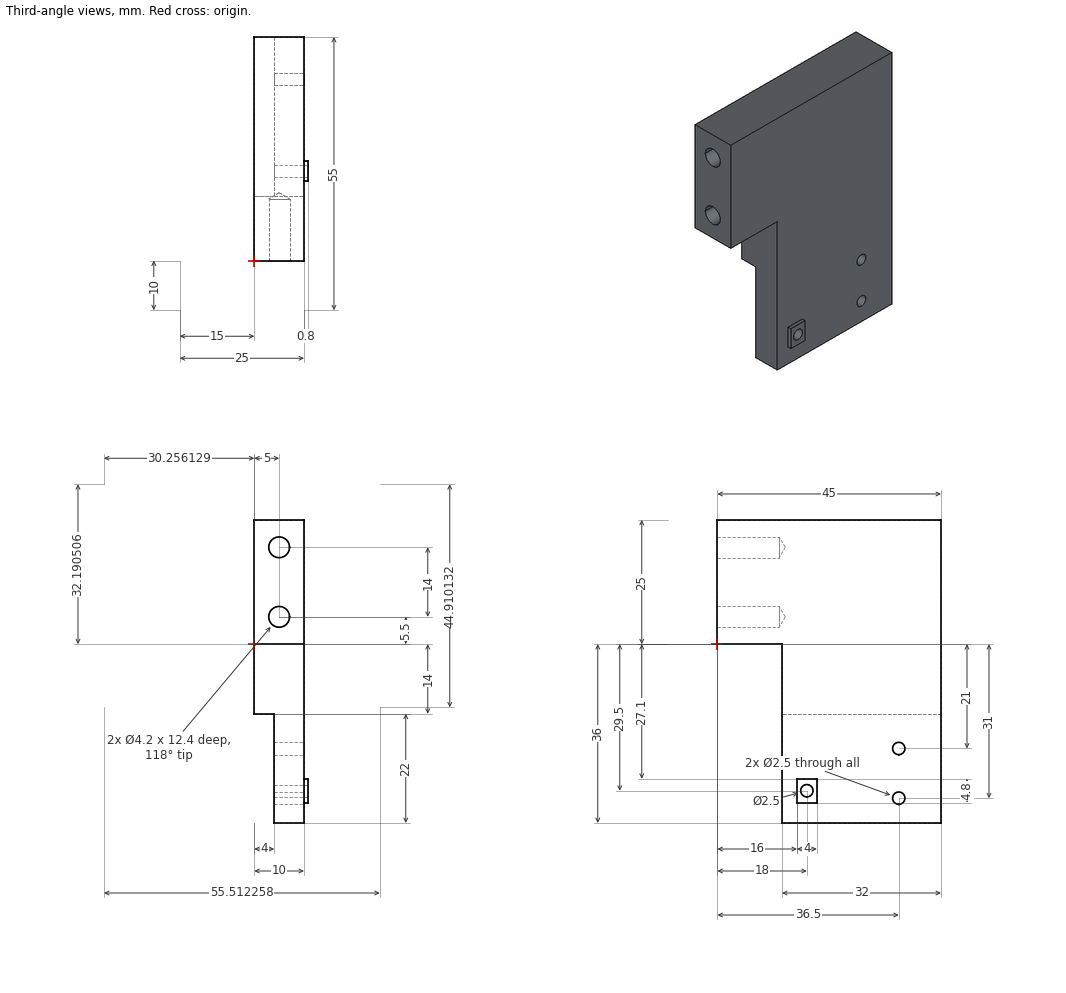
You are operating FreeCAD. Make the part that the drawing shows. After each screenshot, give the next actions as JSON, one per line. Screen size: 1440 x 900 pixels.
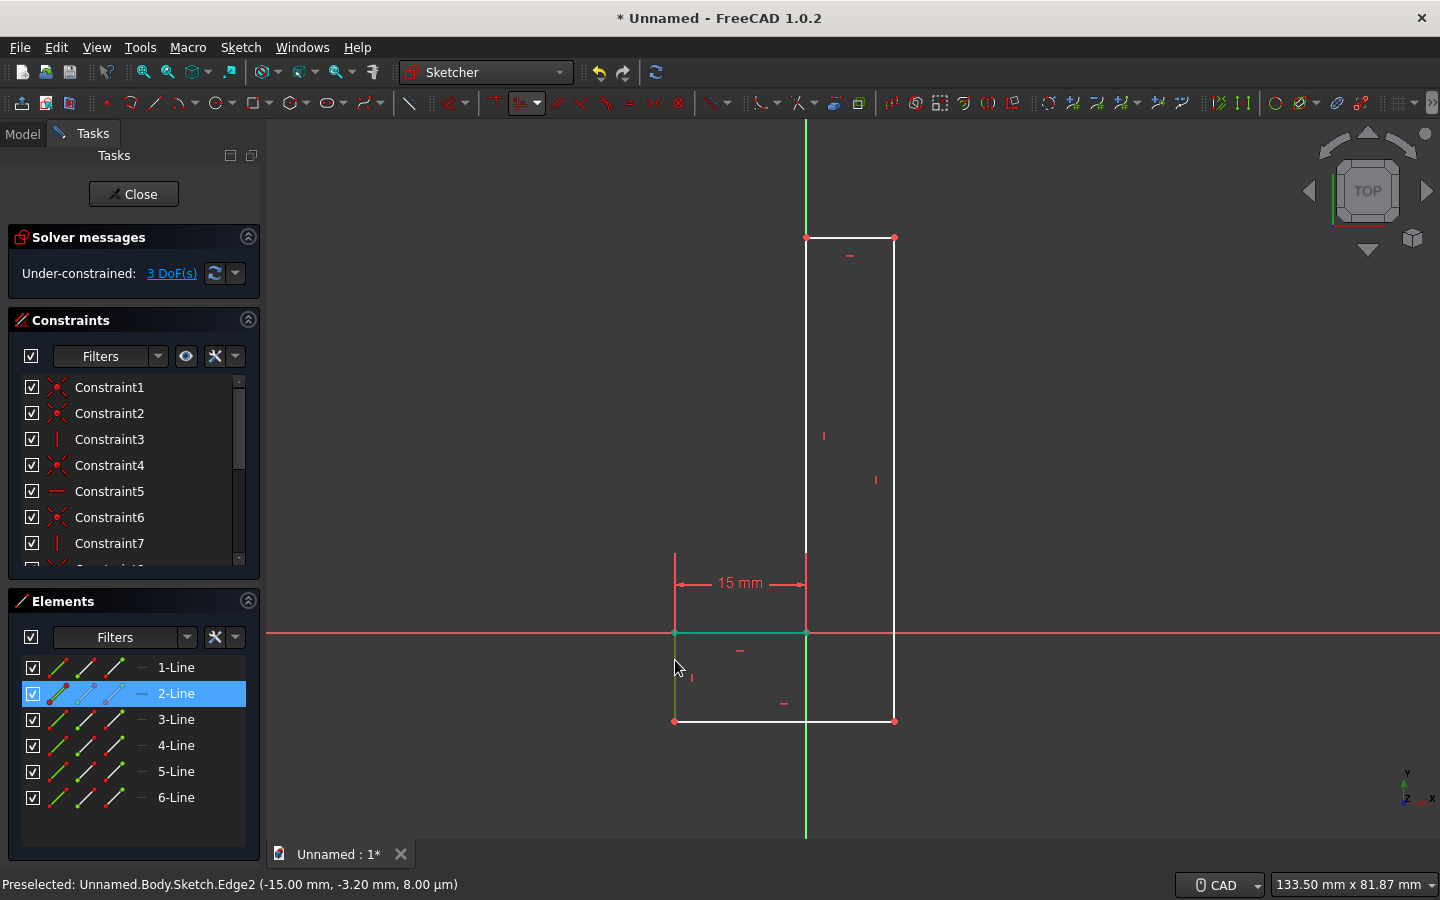
{"action": "key", "text": "i"}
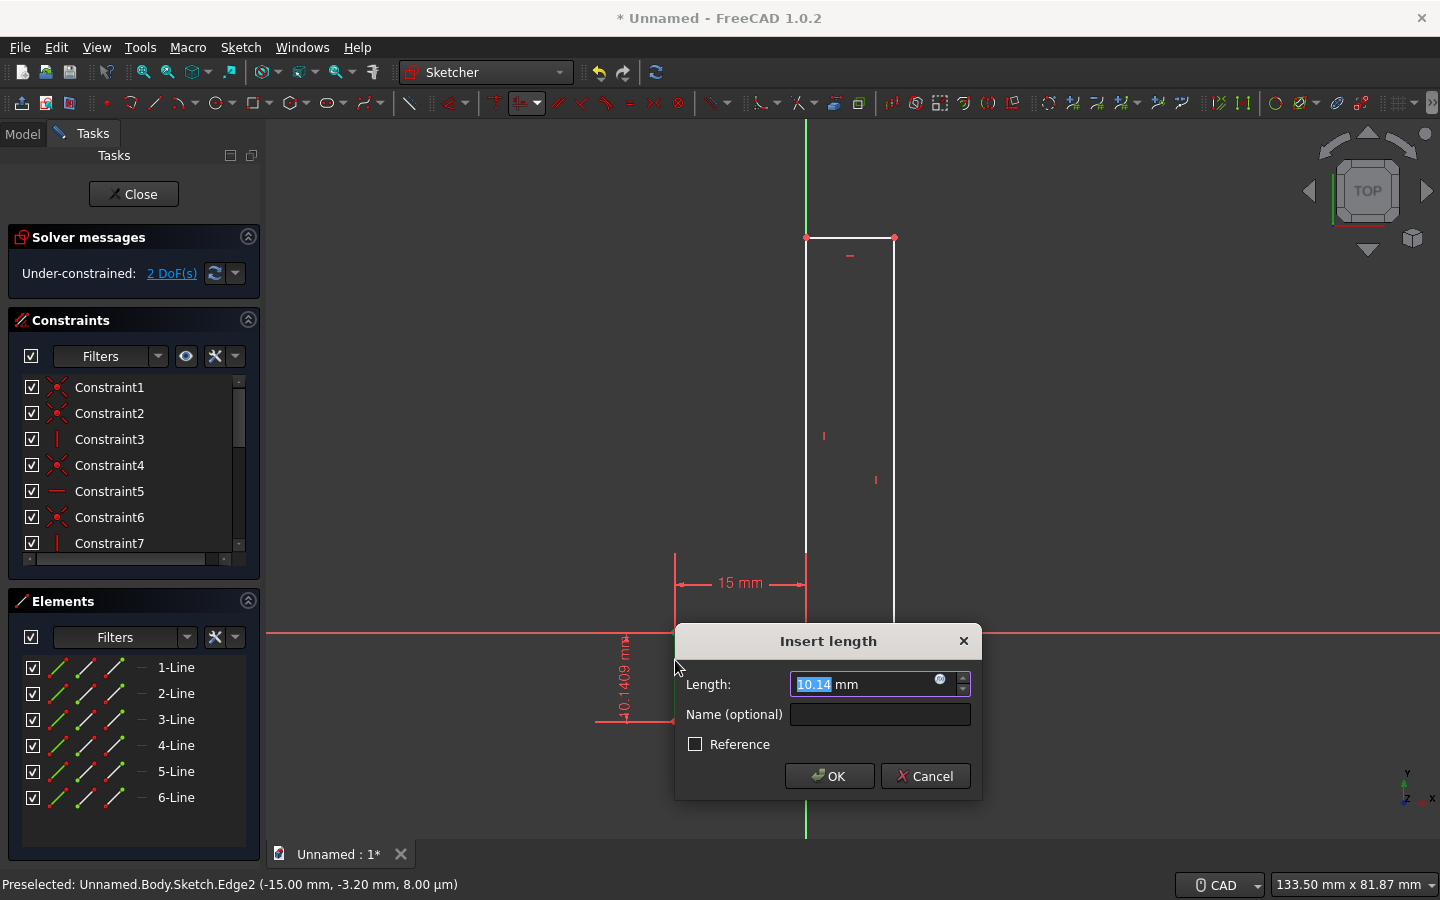
{"action": "type", "text": "10"}
{"action": "key", "text": "Return"}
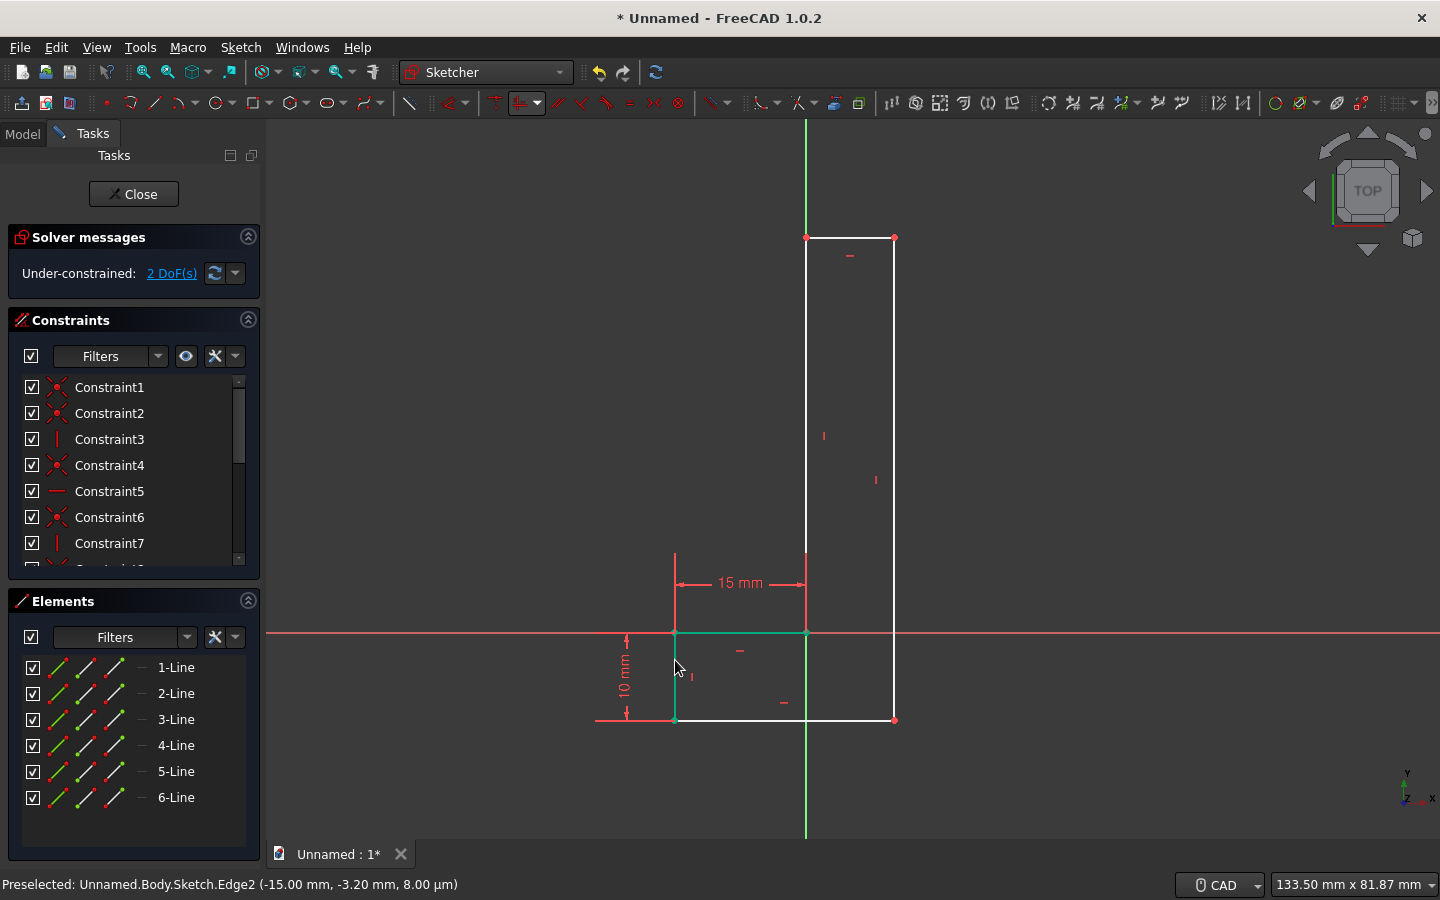
{"action": "left_click", "coordinate": [740, 721]}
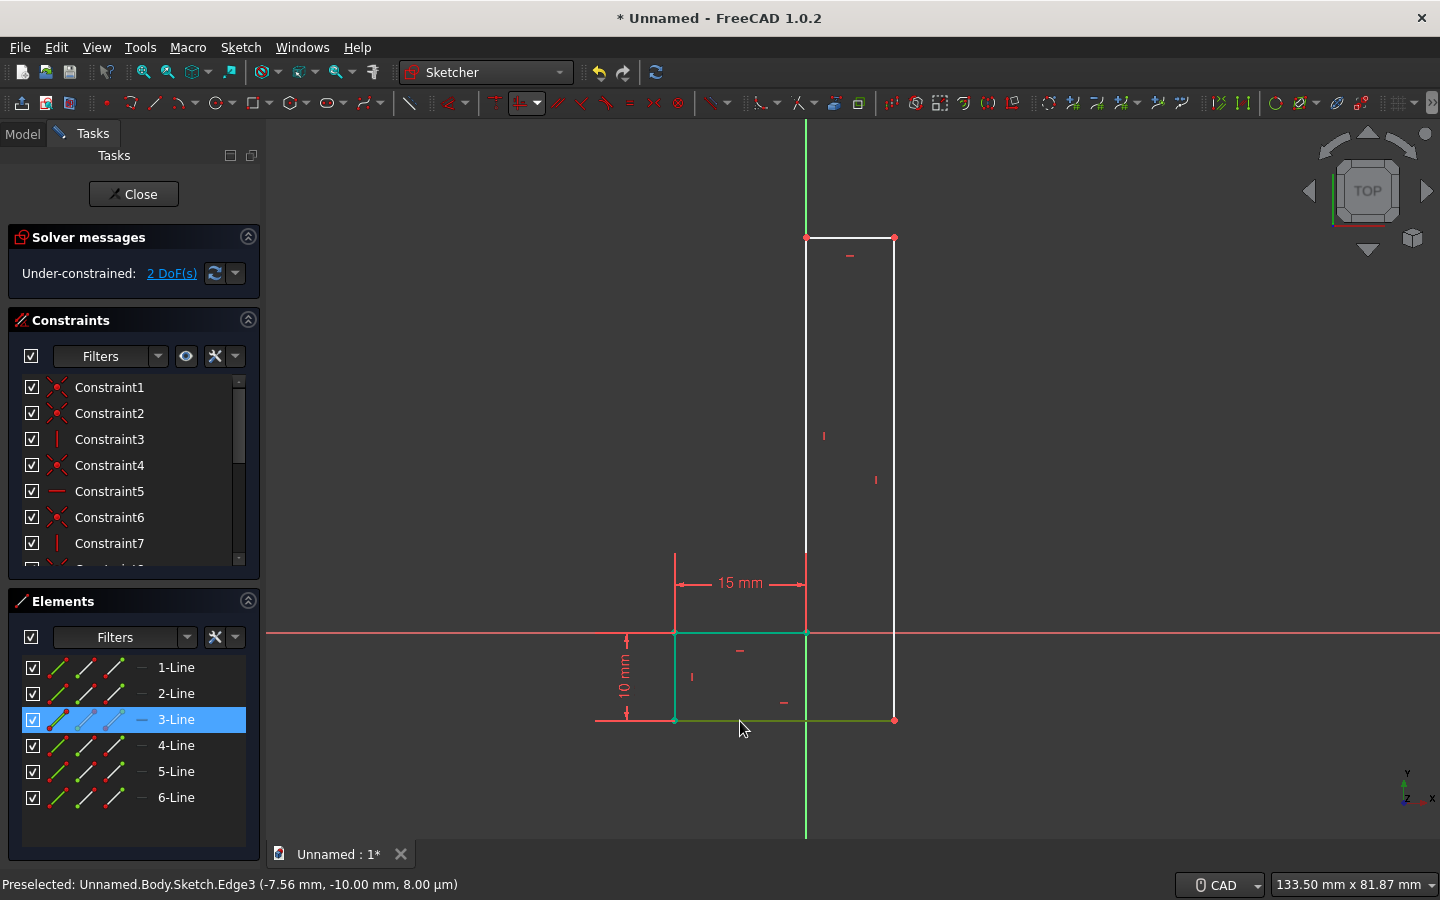
{"action": "key", "text": "l"}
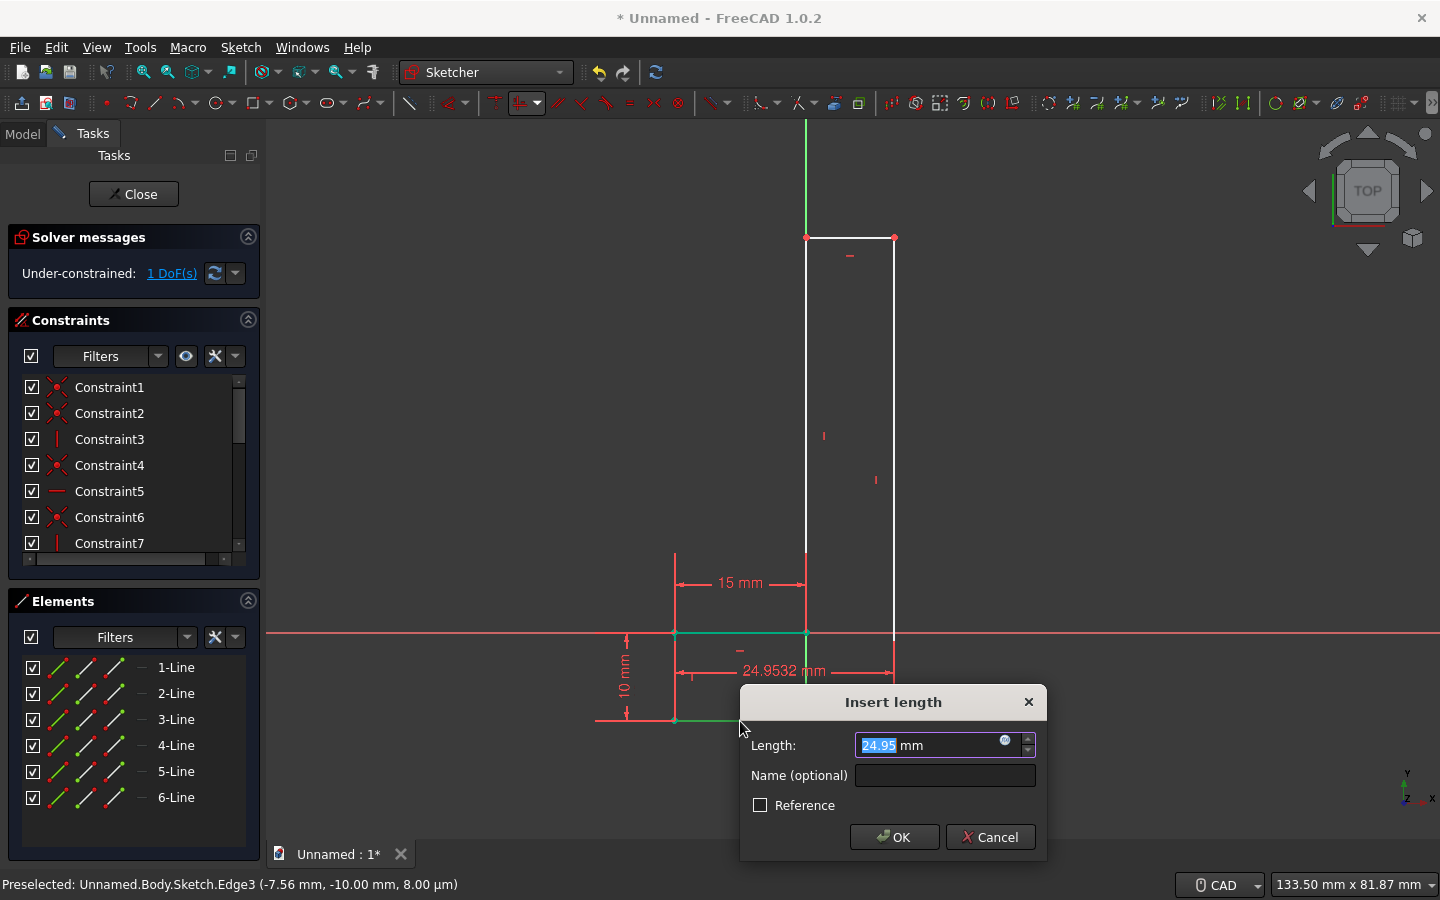
{"action": "type", "text": "25"}
{"action": "key", "text": "Return"}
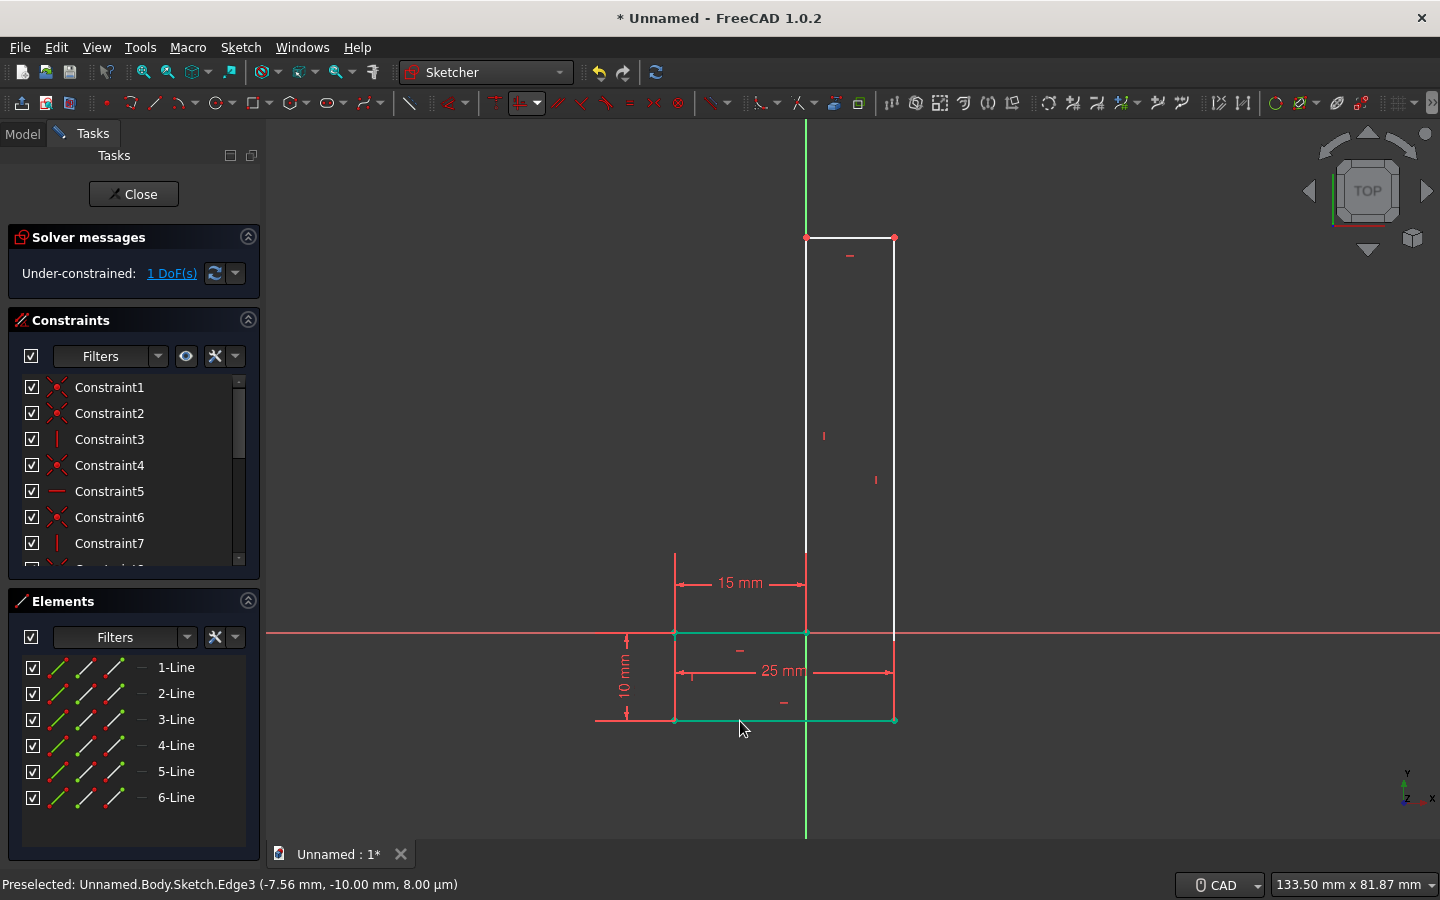
{"action": "left_click", "coordinate": [894, 576]}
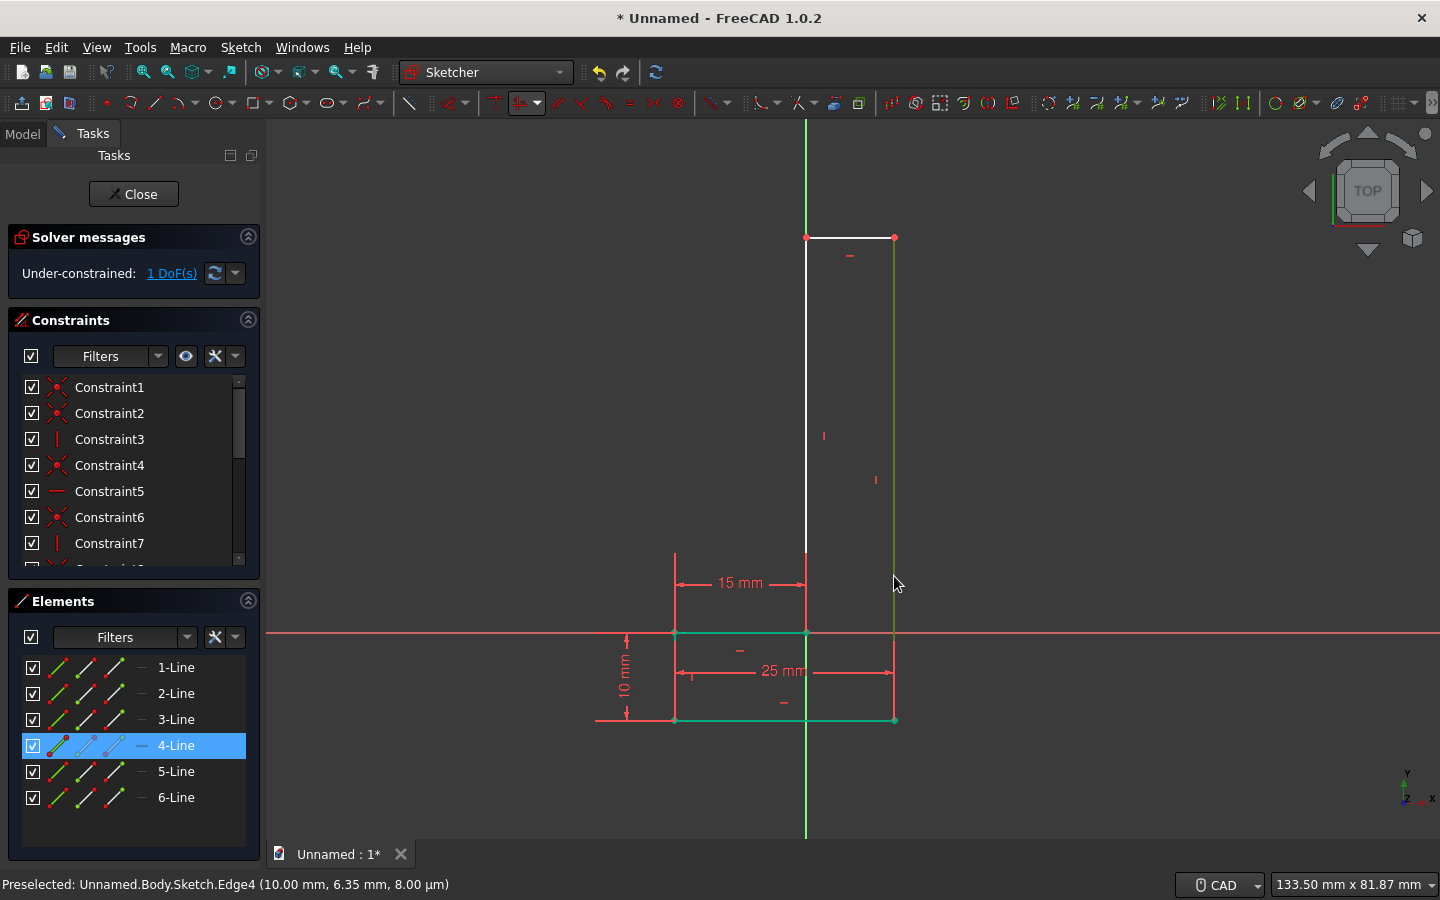
{"action": "key", "text": "i"}